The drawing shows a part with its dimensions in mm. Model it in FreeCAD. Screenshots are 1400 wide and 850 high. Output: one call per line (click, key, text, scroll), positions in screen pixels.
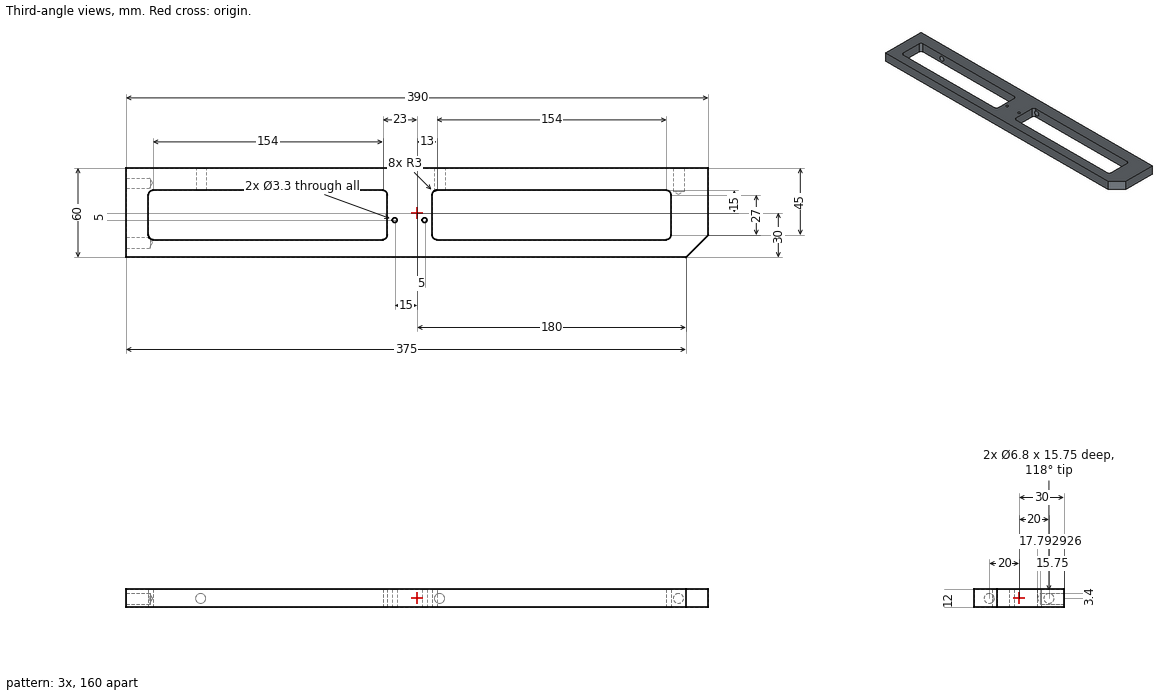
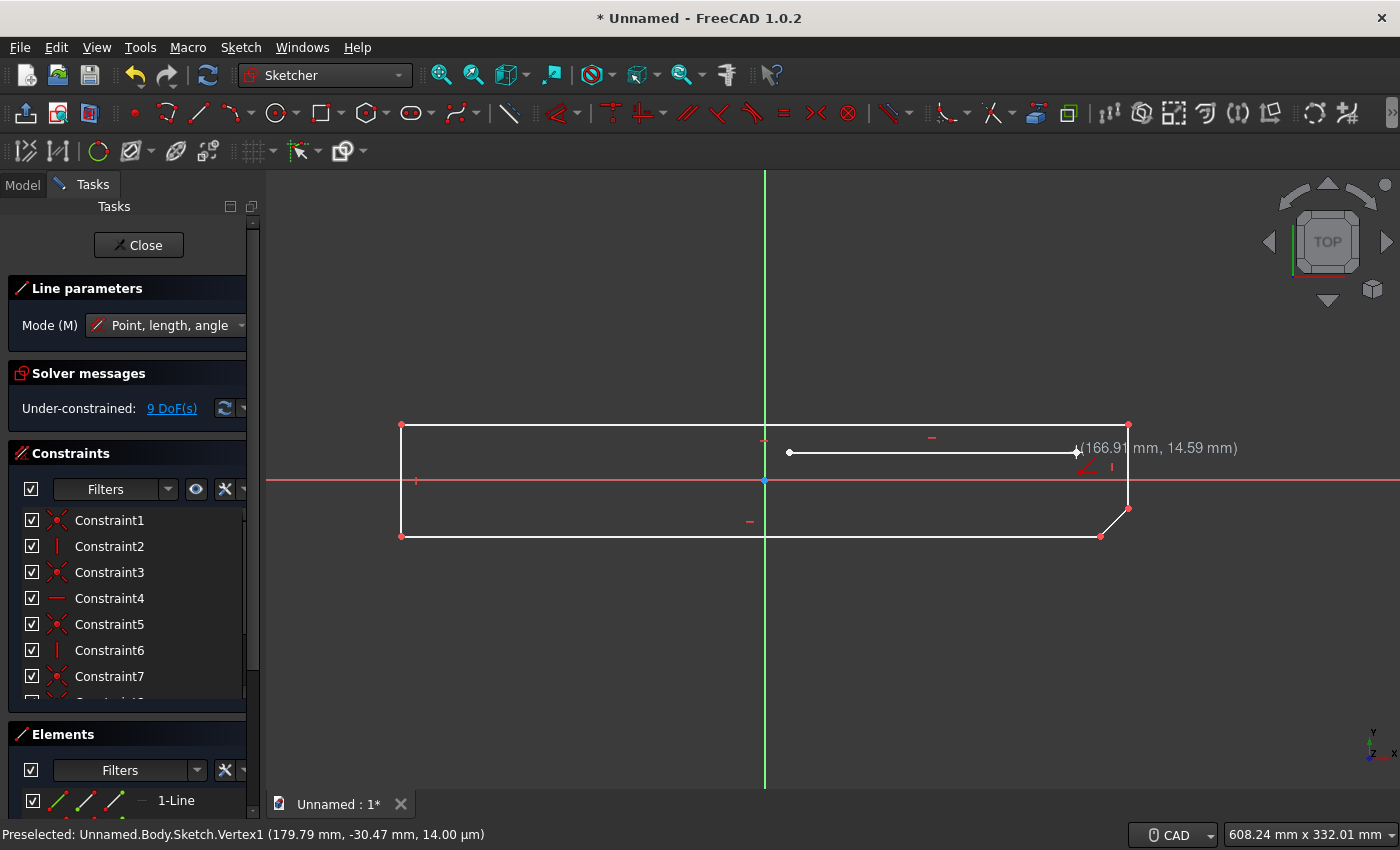
scroll(1082, 458, up, 4)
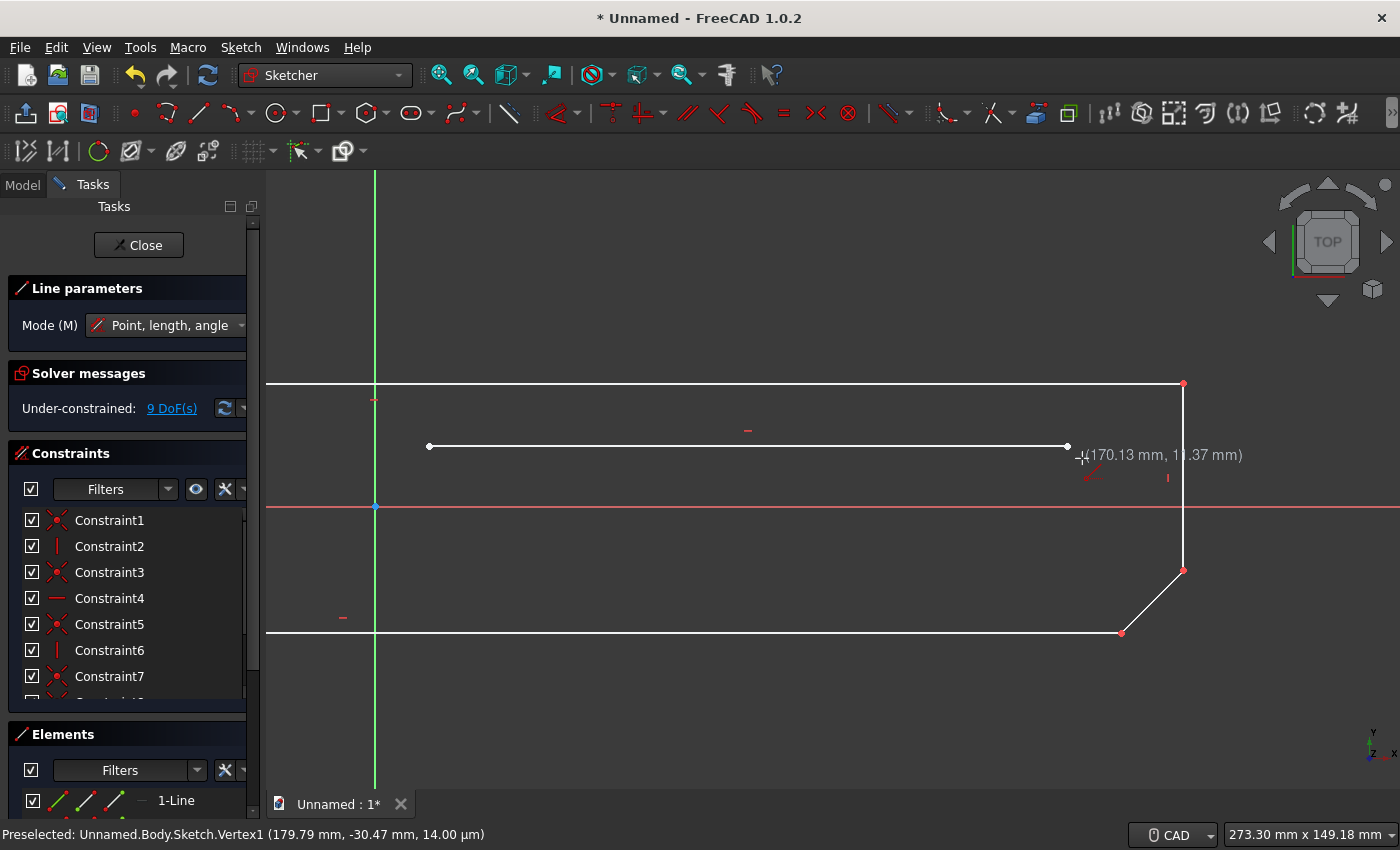
click(1081, 457)
click(1081, 569)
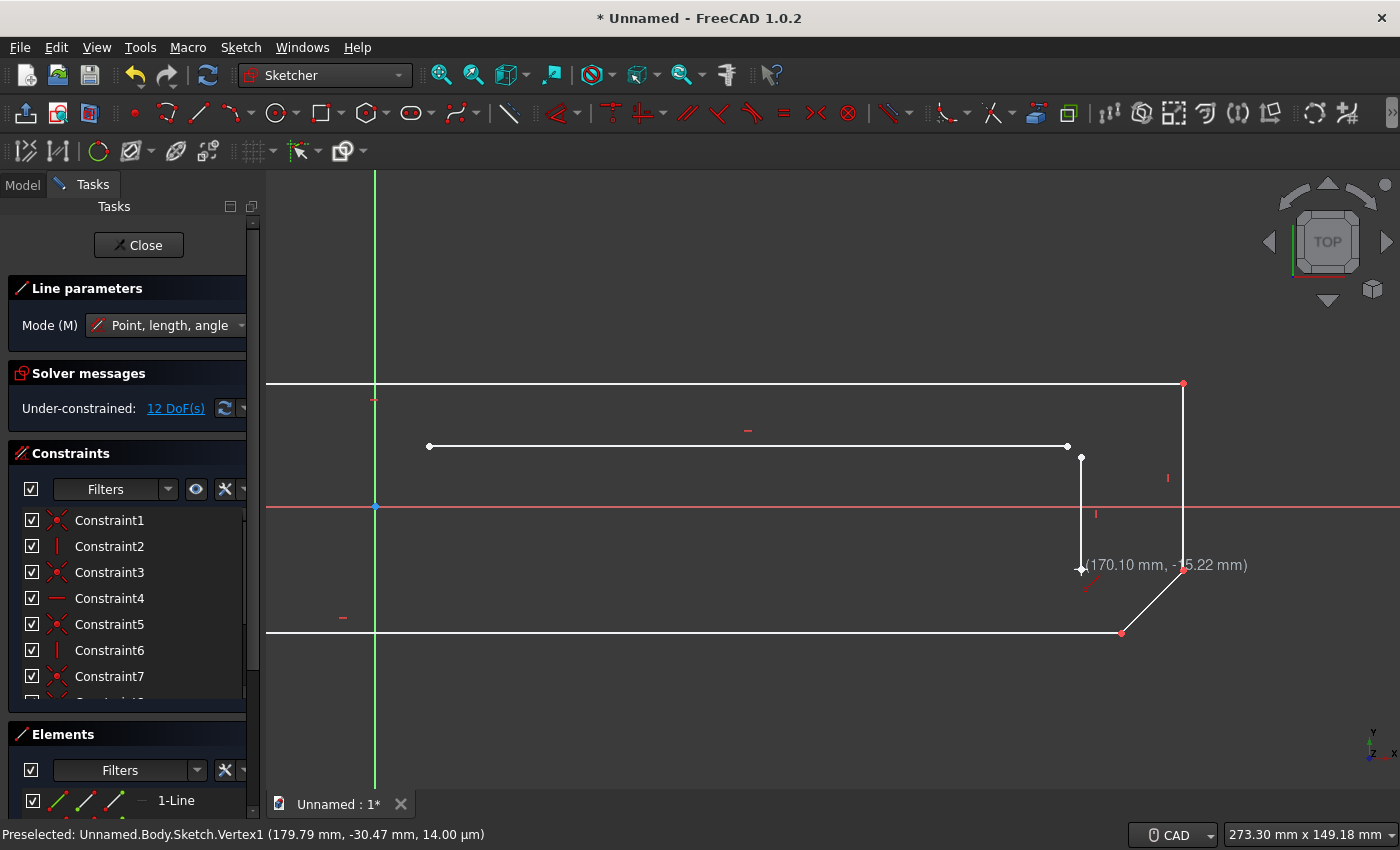
click(1068, 582)
click(429, 582)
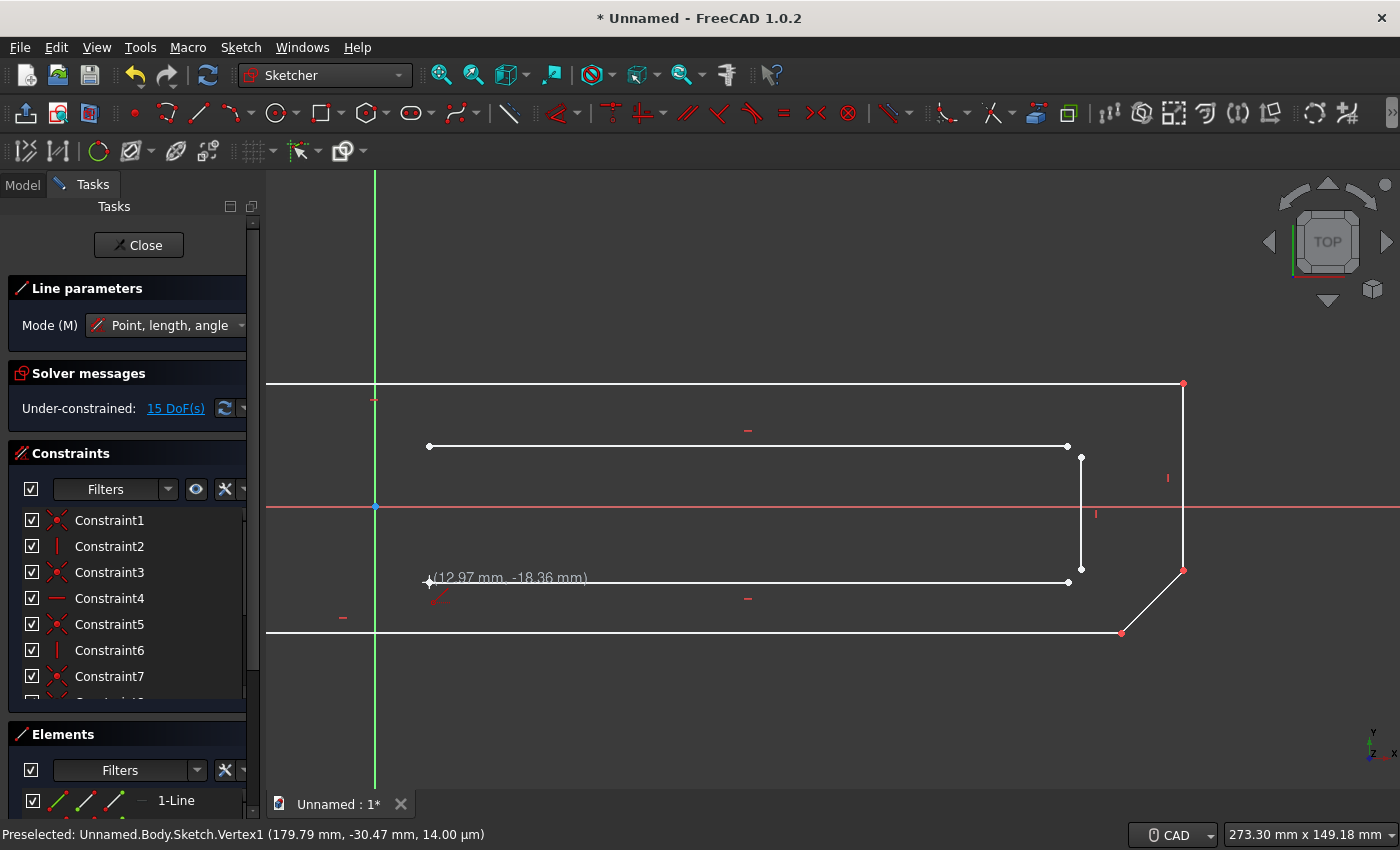
click(417, 569)
click(417, 457)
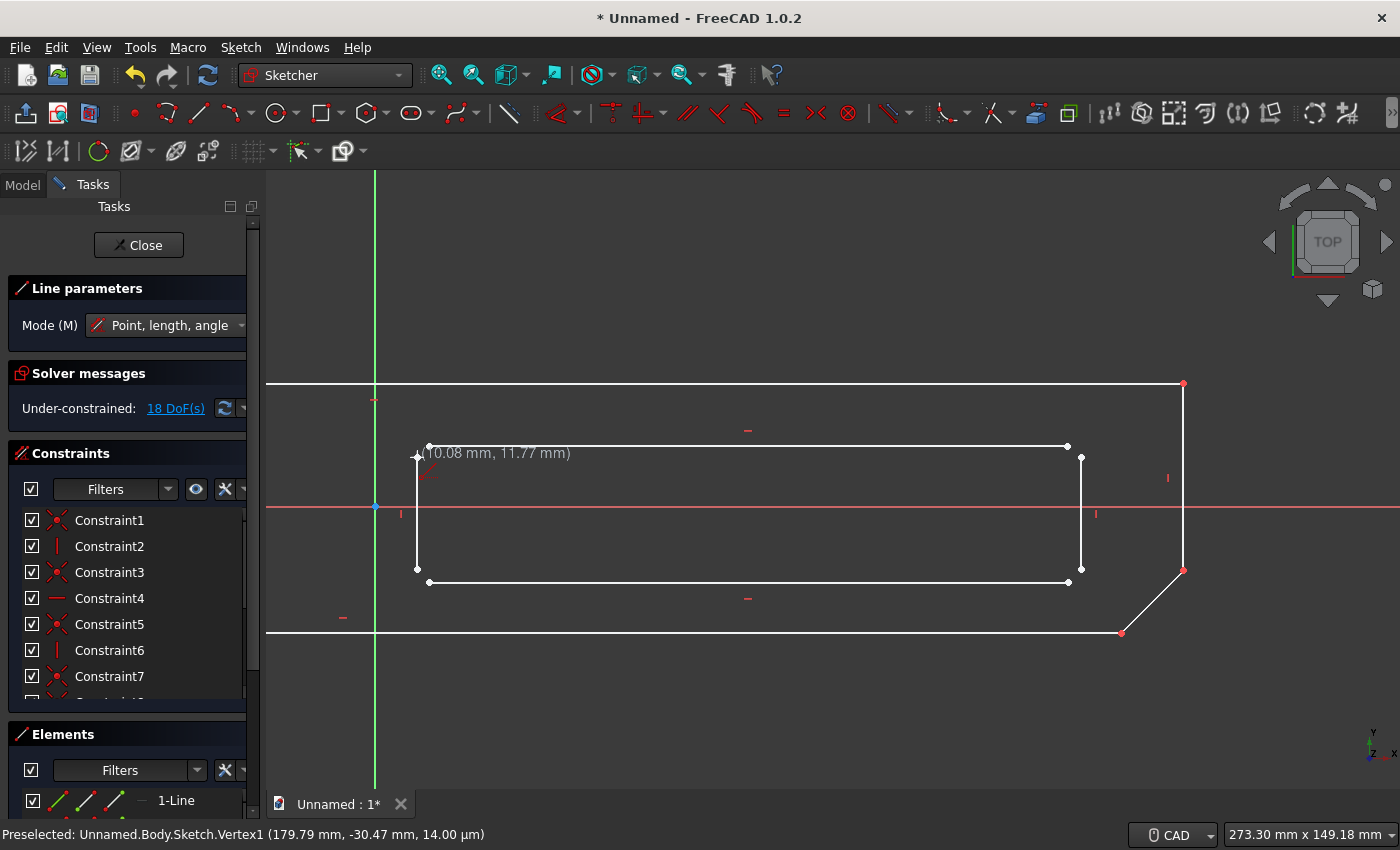
click(232, 114)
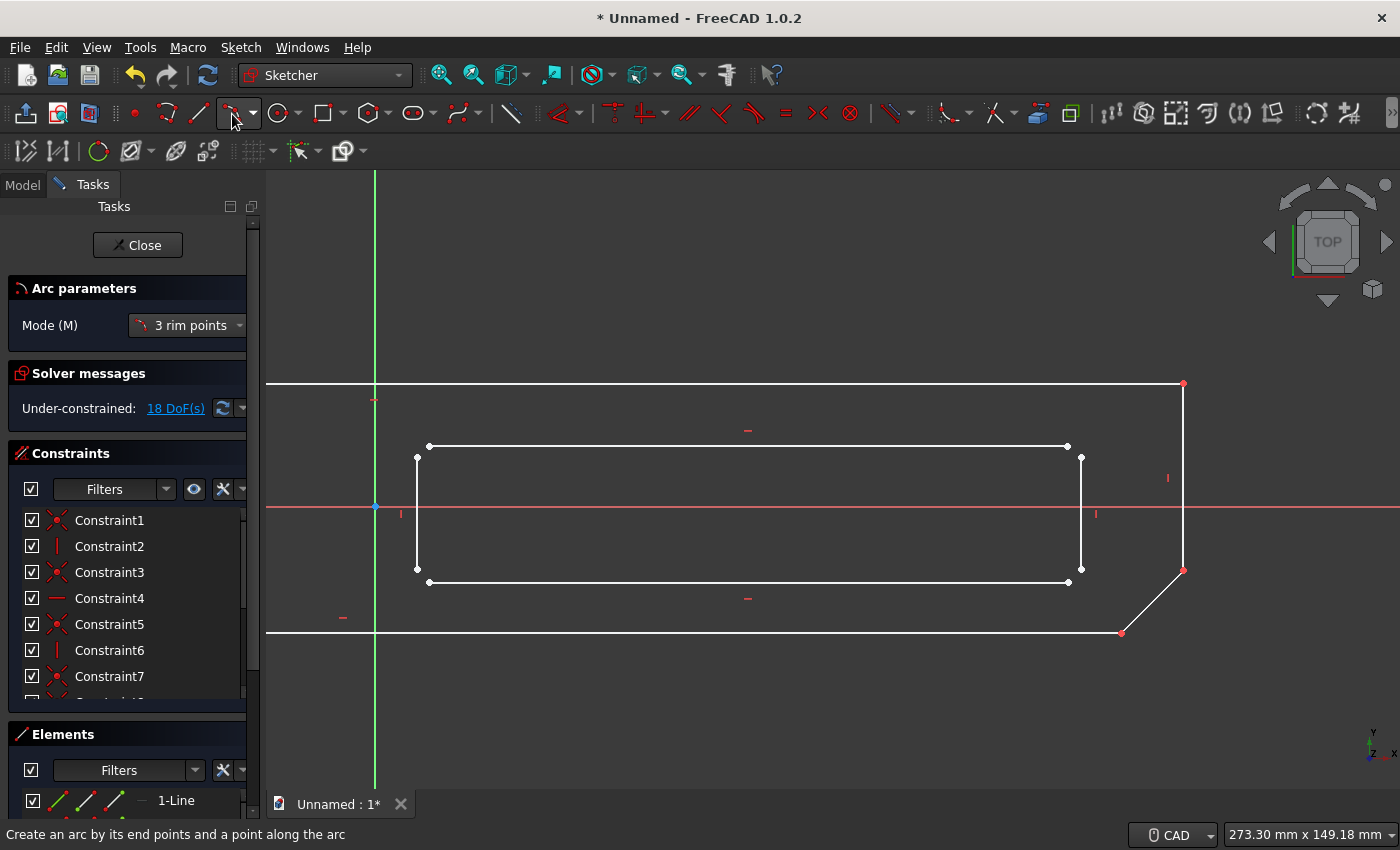
click(1068, 446)
click(1081, 458)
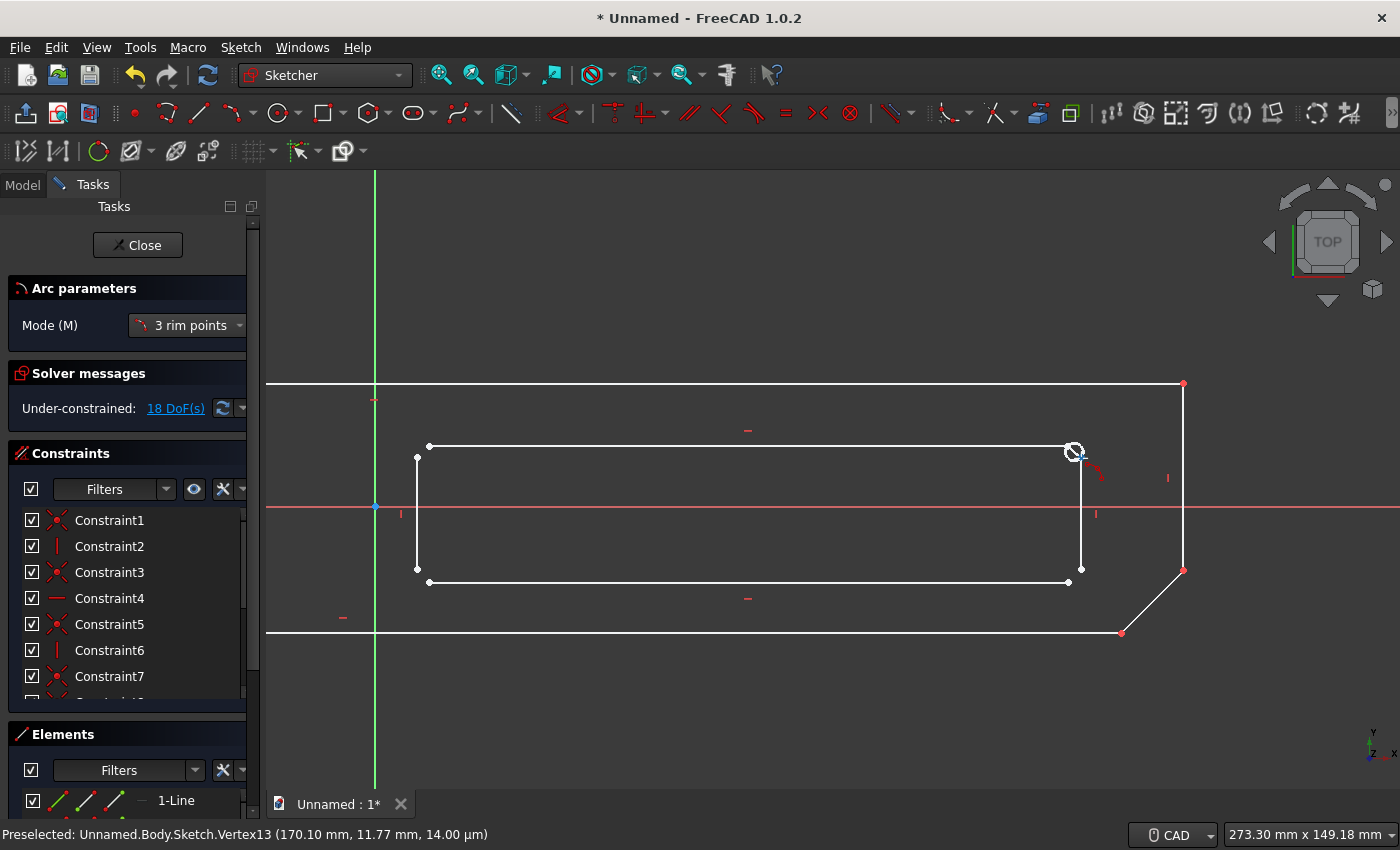
scroll(1077, 448, up, 8)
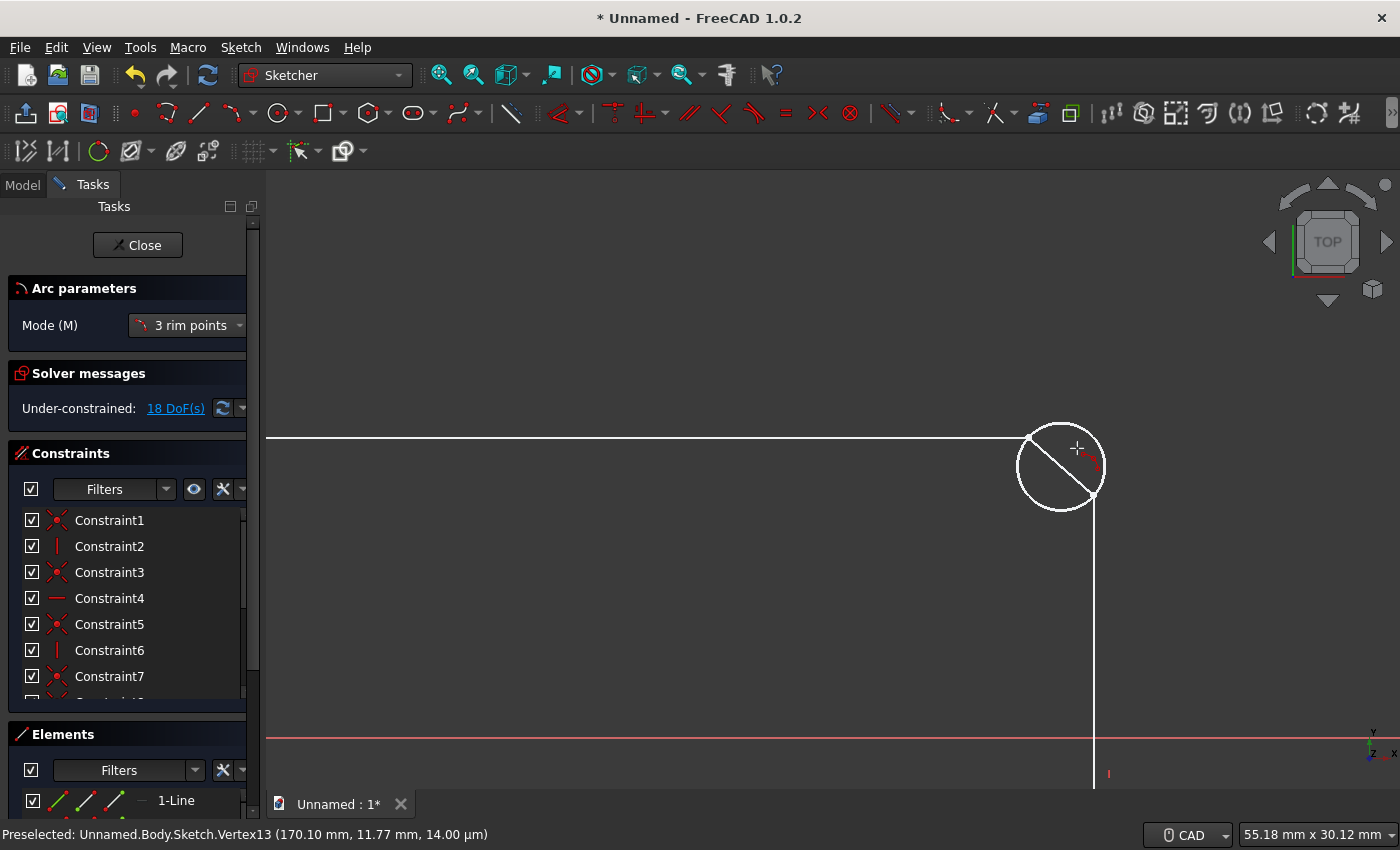
click(1074, 447)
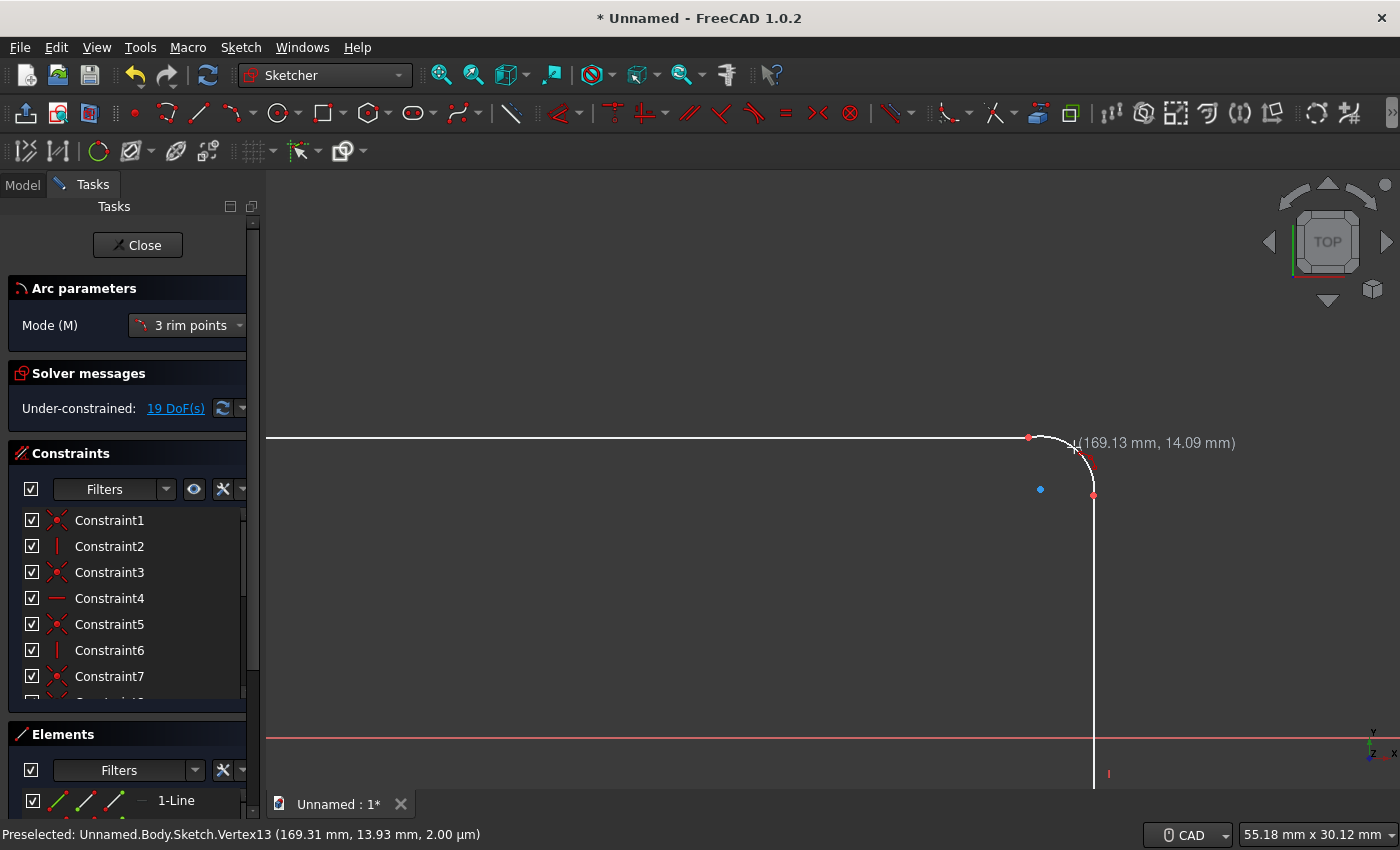
scroll(1080, 454, down, 12)